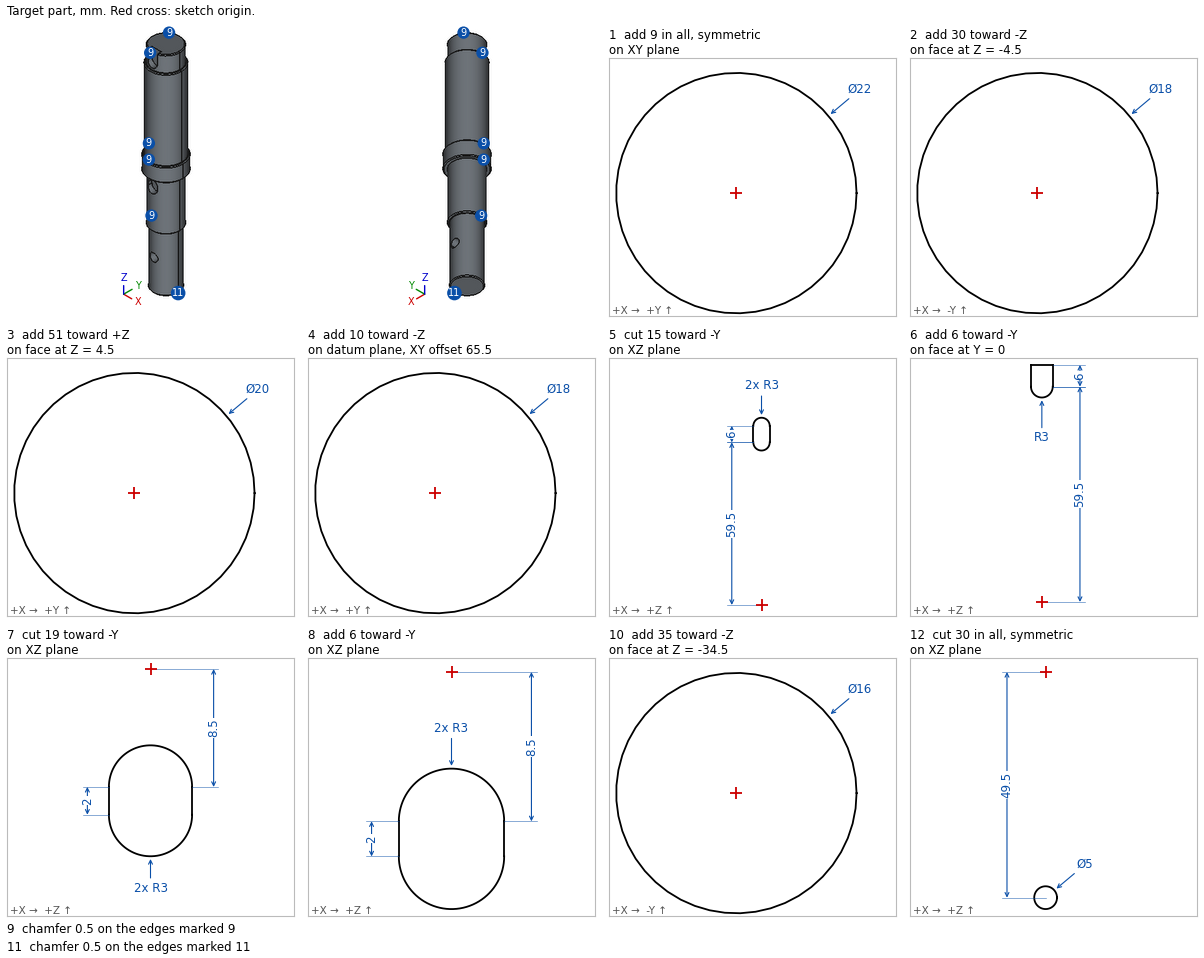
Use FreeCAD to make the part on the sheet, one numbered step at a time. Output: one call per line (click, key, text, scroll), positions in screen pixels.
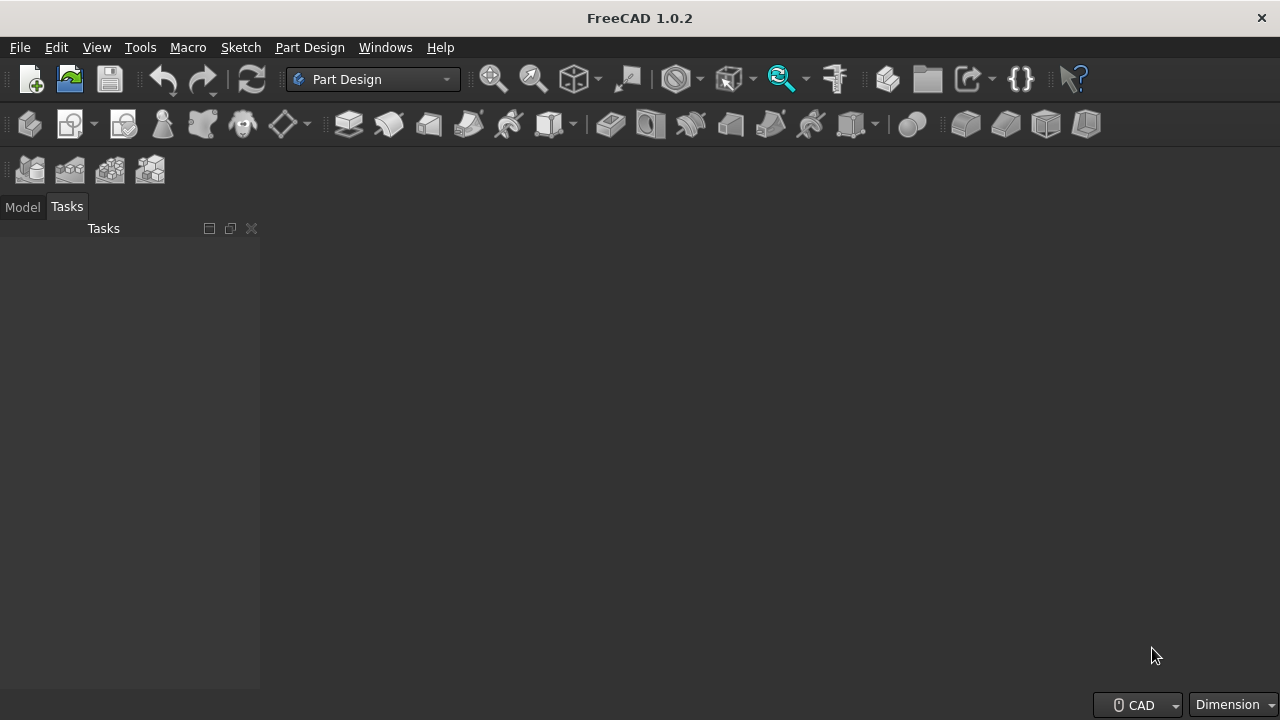
click(30, 80)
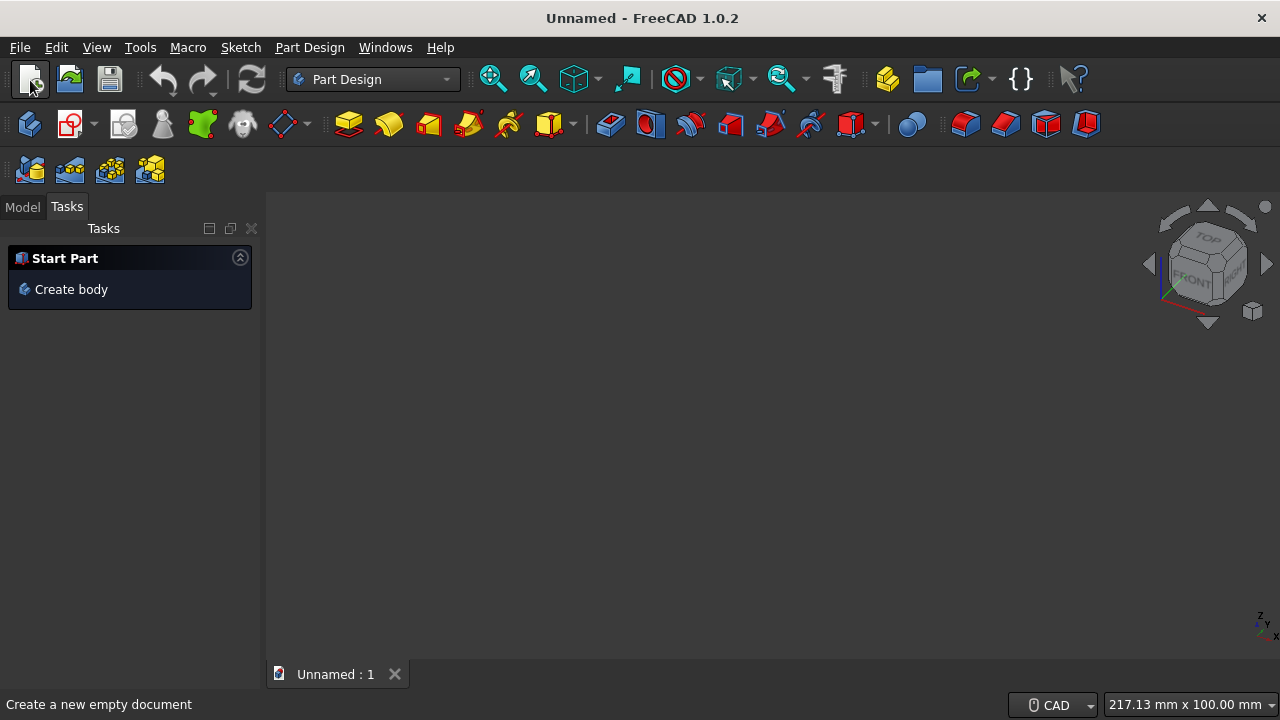
click(70, 124)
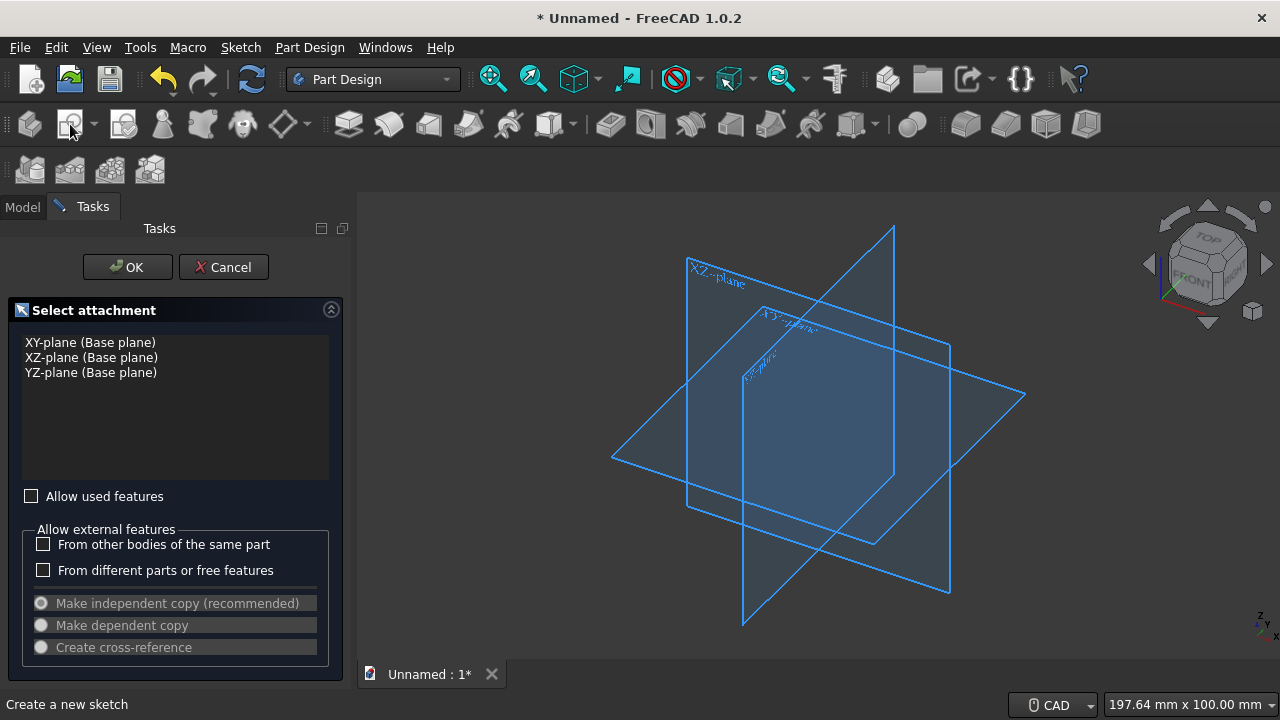
click(82, 342)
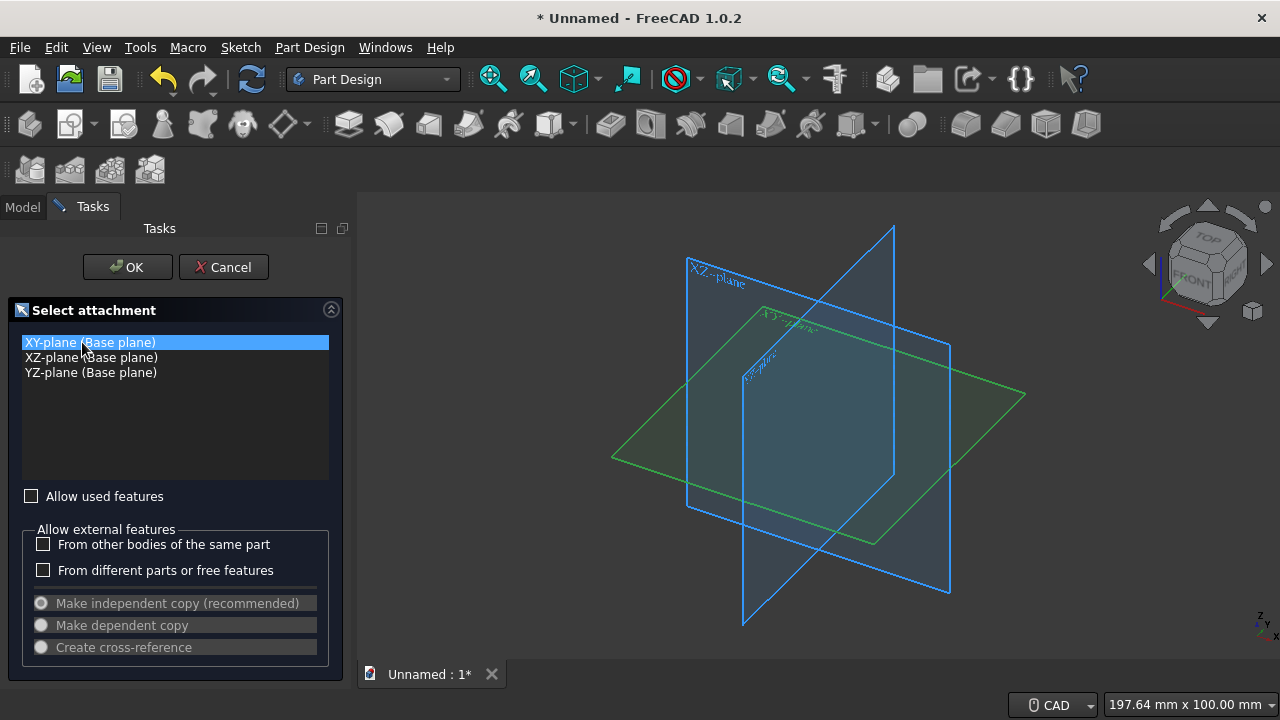
click(128, 267)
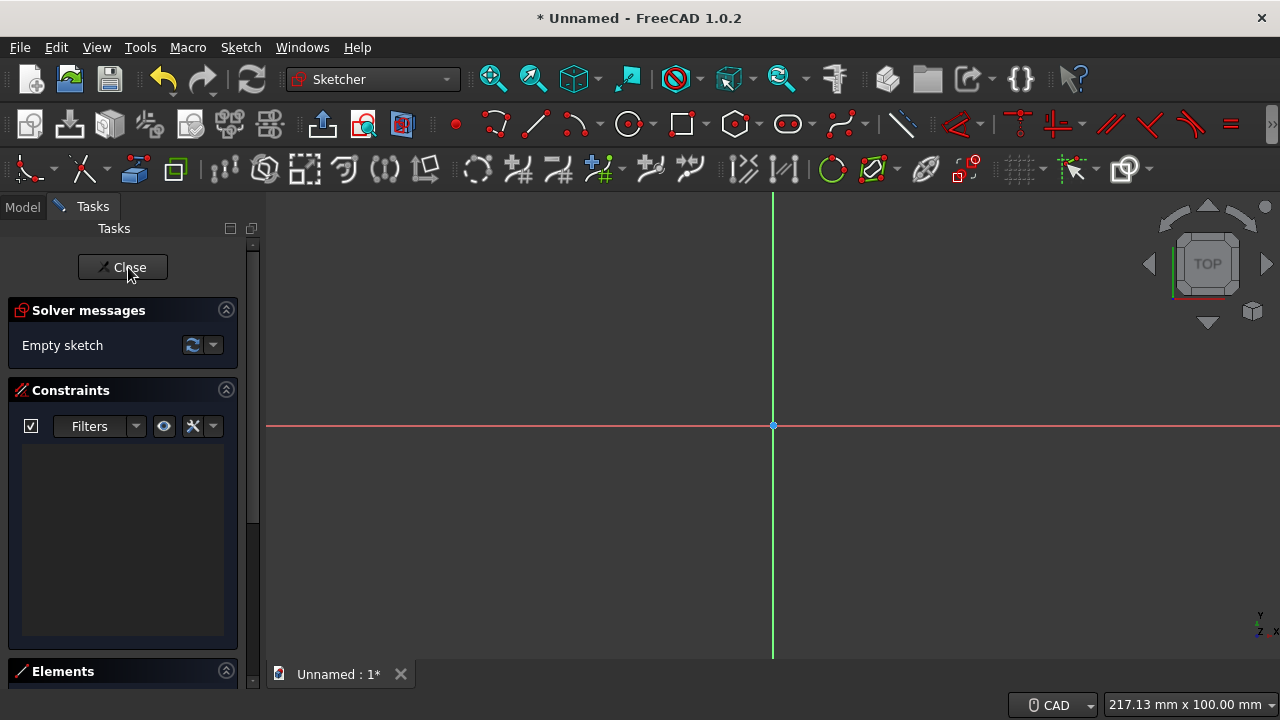
scroll(813, 426, up, 5)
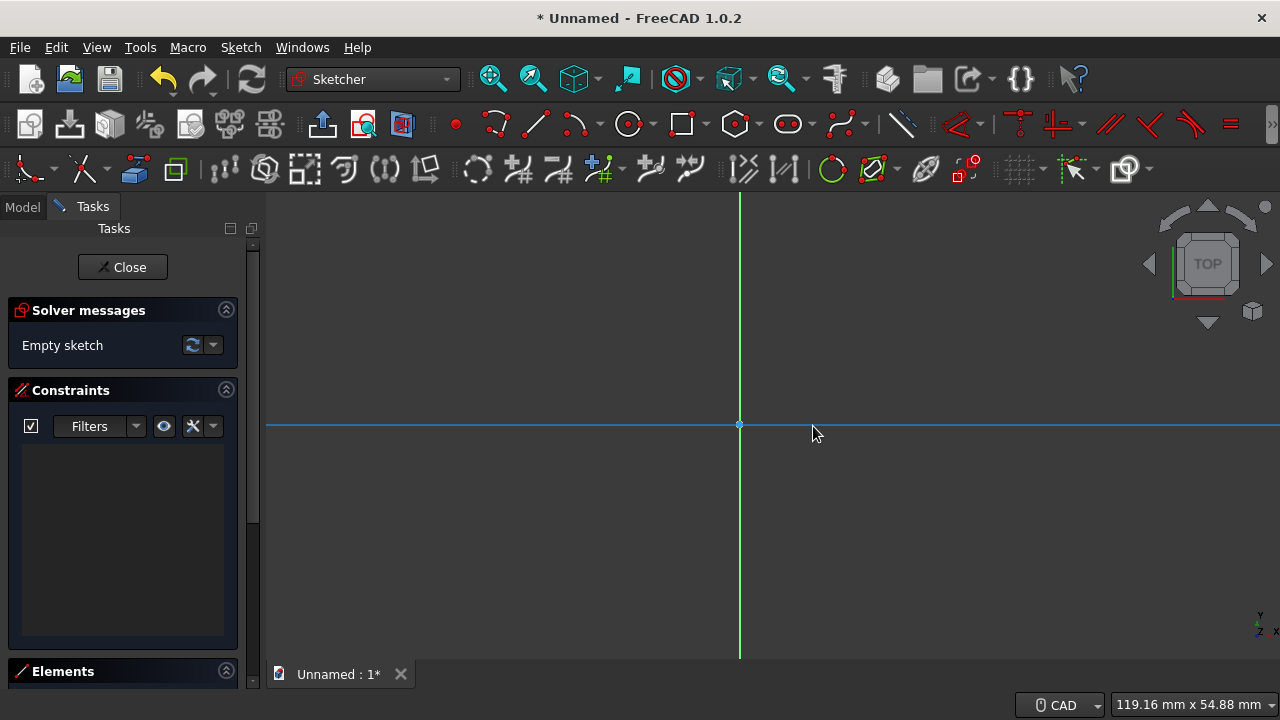
click(630, 124)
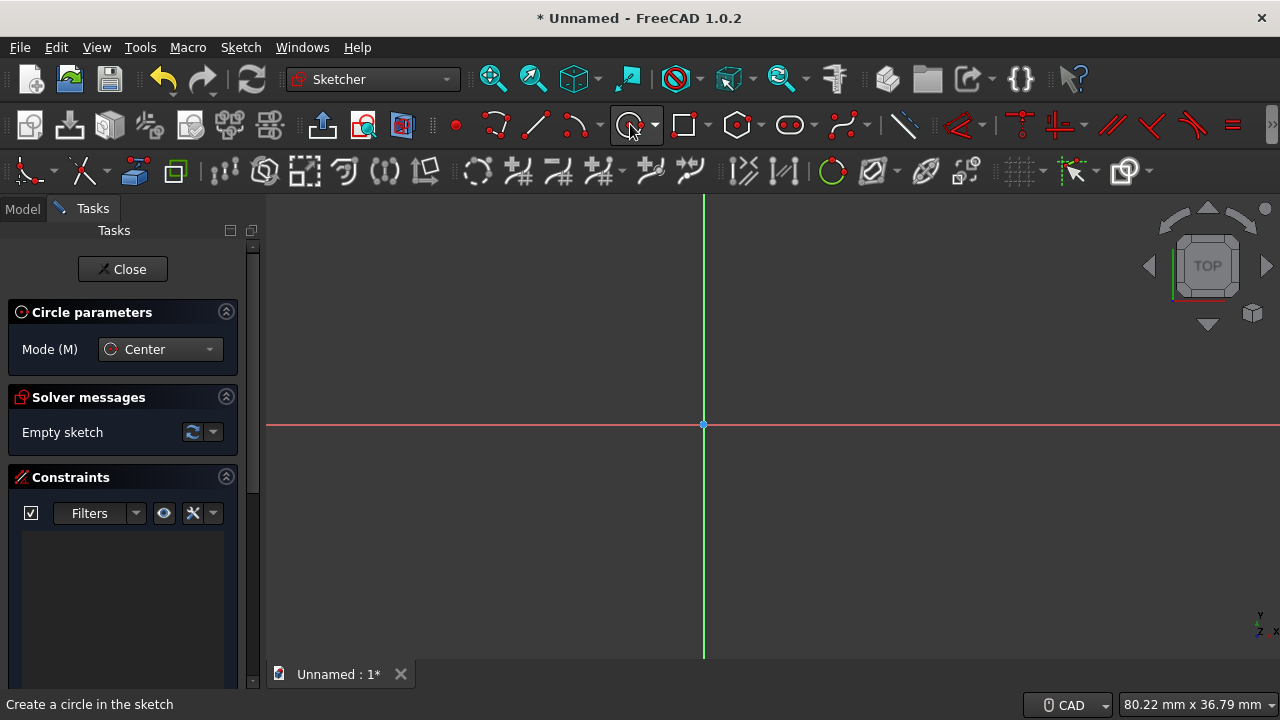
click(704, 425)
click(802, 326)
key(Escape)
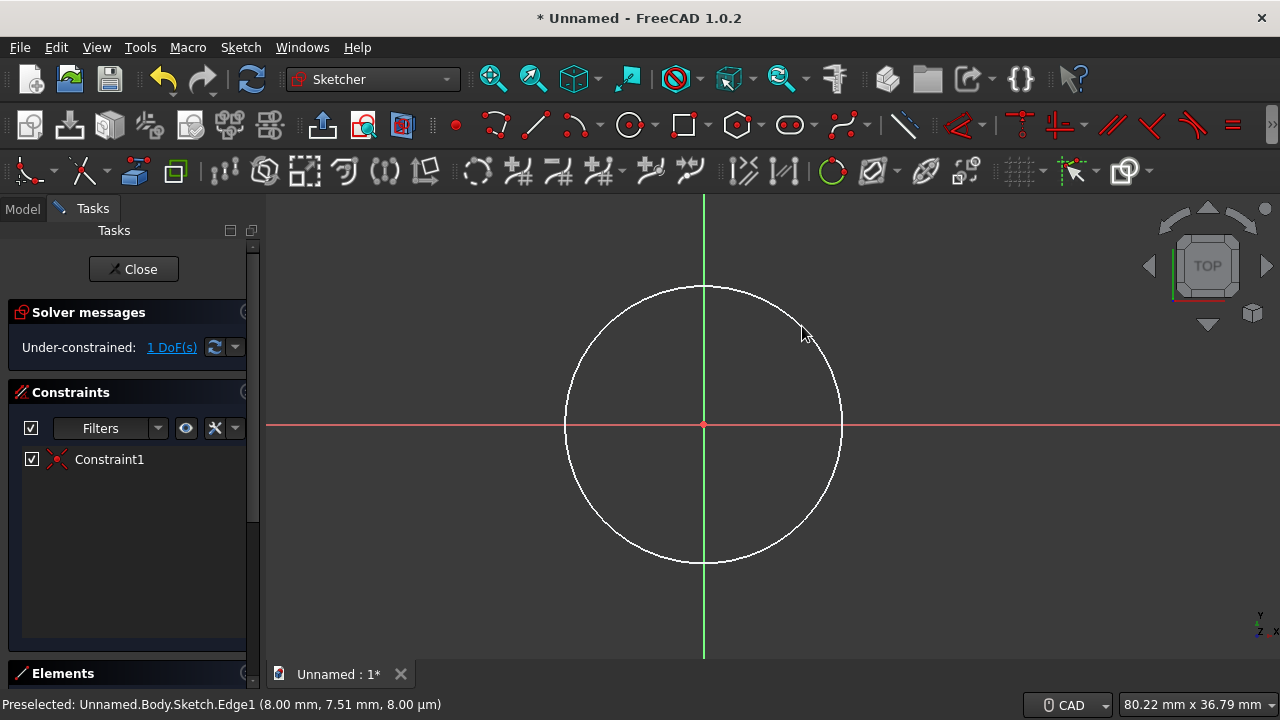
click(801, 326)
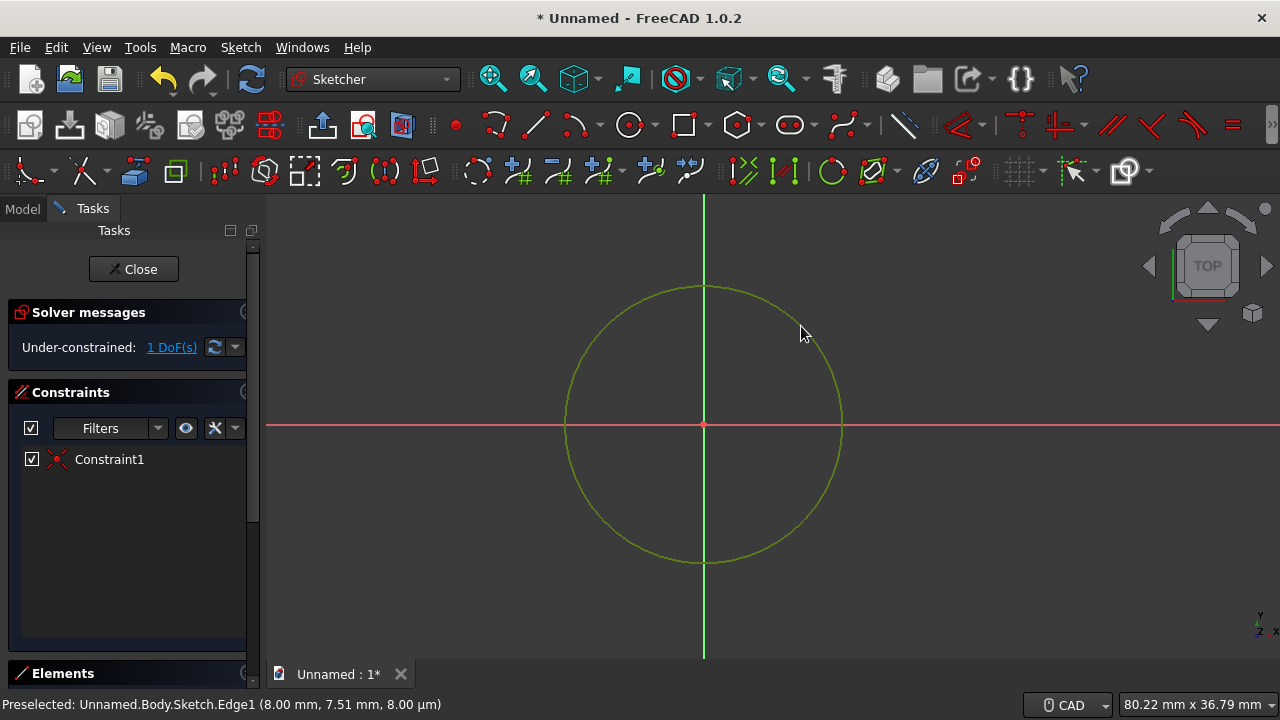
click(984, 126)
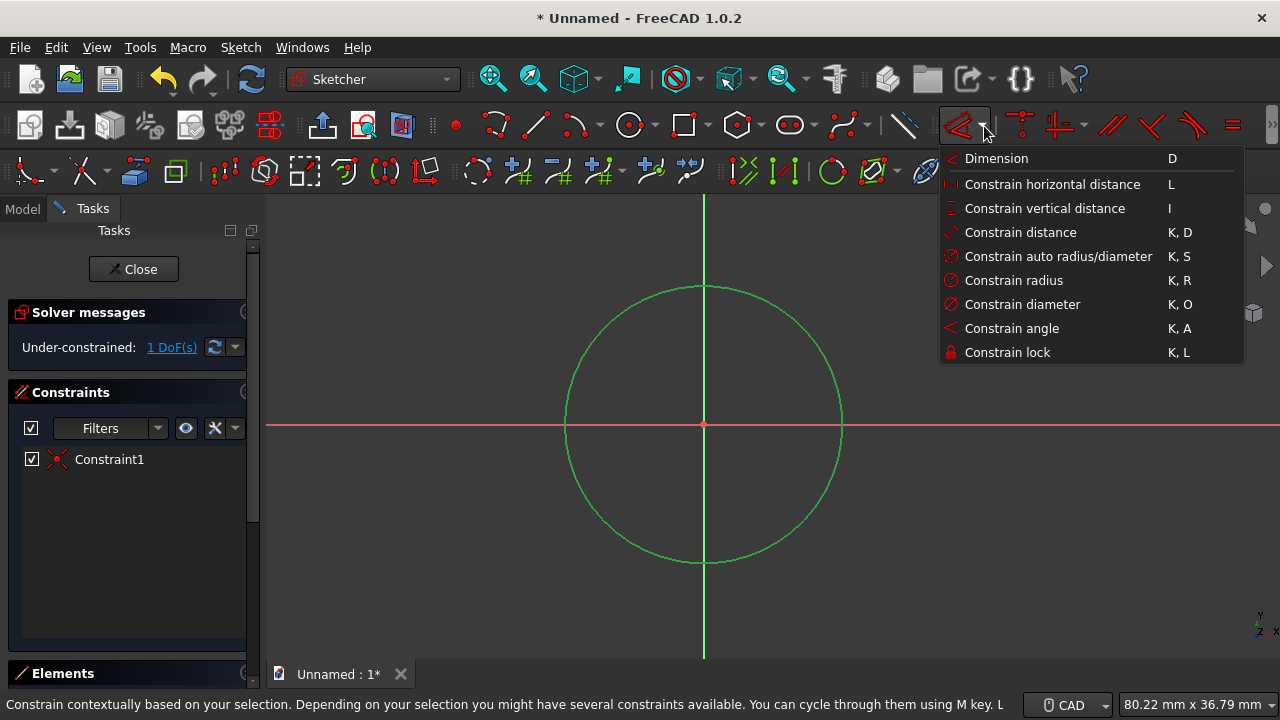
click(1092, 304)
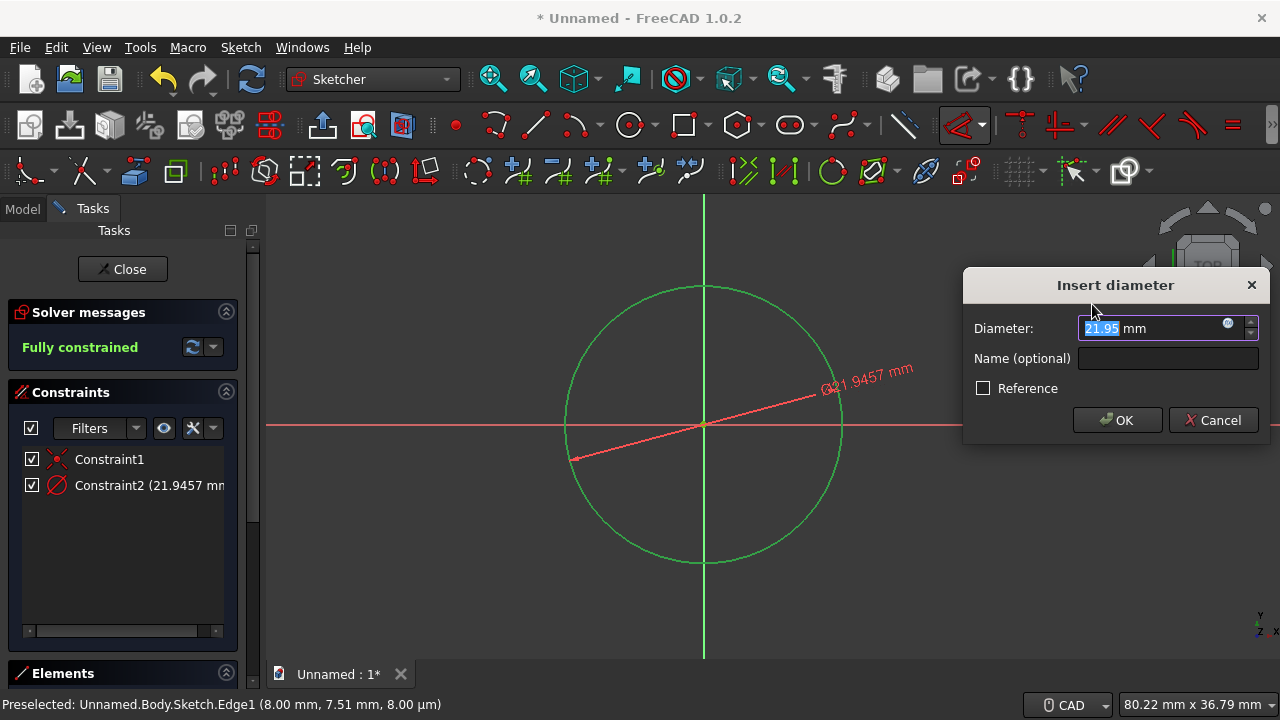
text(22)
key(Return)